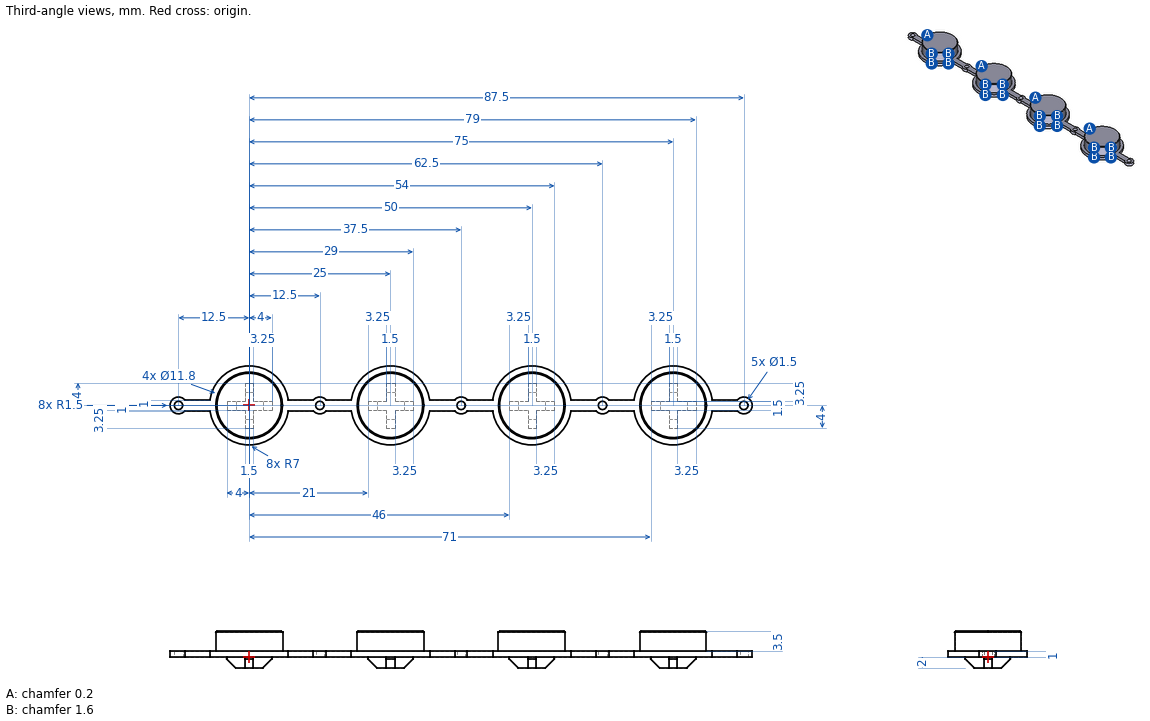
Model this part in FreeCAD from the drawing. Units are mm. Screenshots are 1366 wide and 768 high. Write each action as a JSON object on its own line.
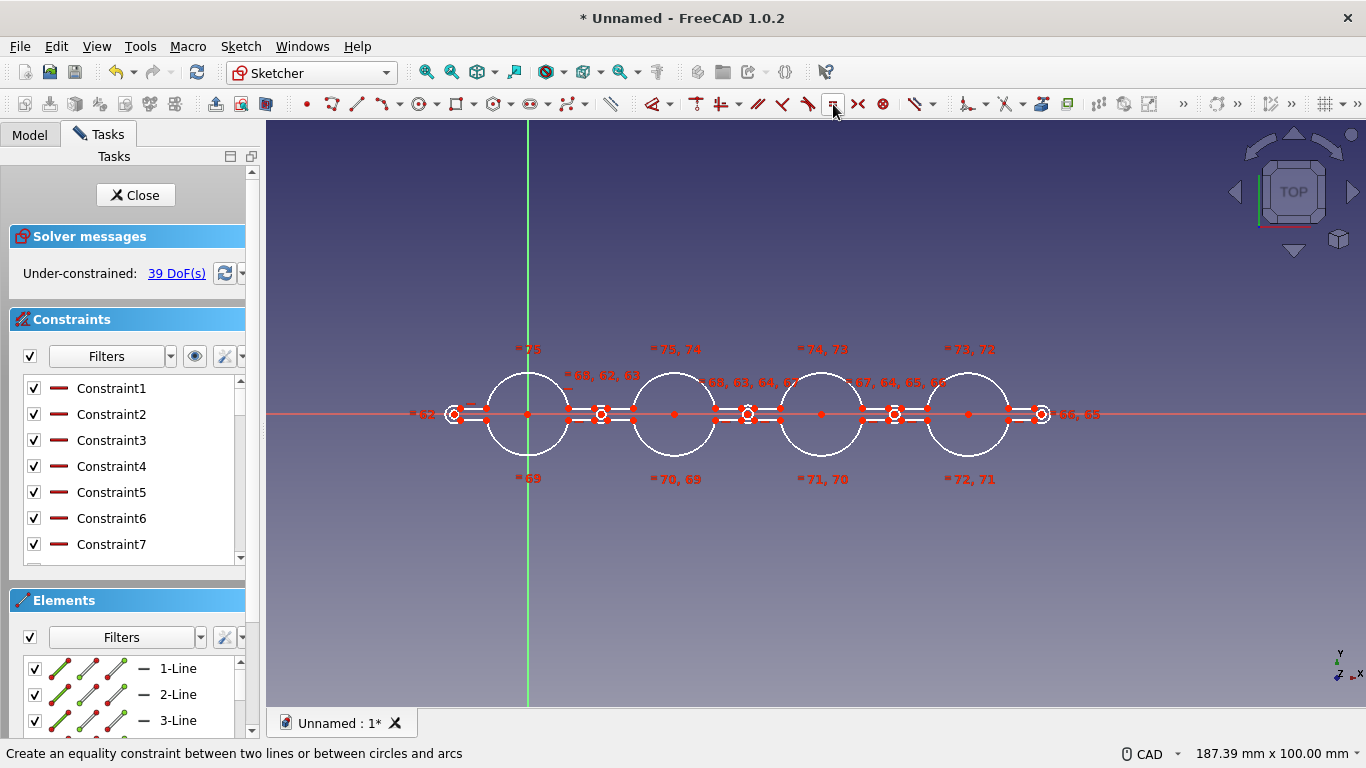
{"action": "scroll", "coordinate": [1037, 414], "scroll_direction": "up", "scroll_amount": 6}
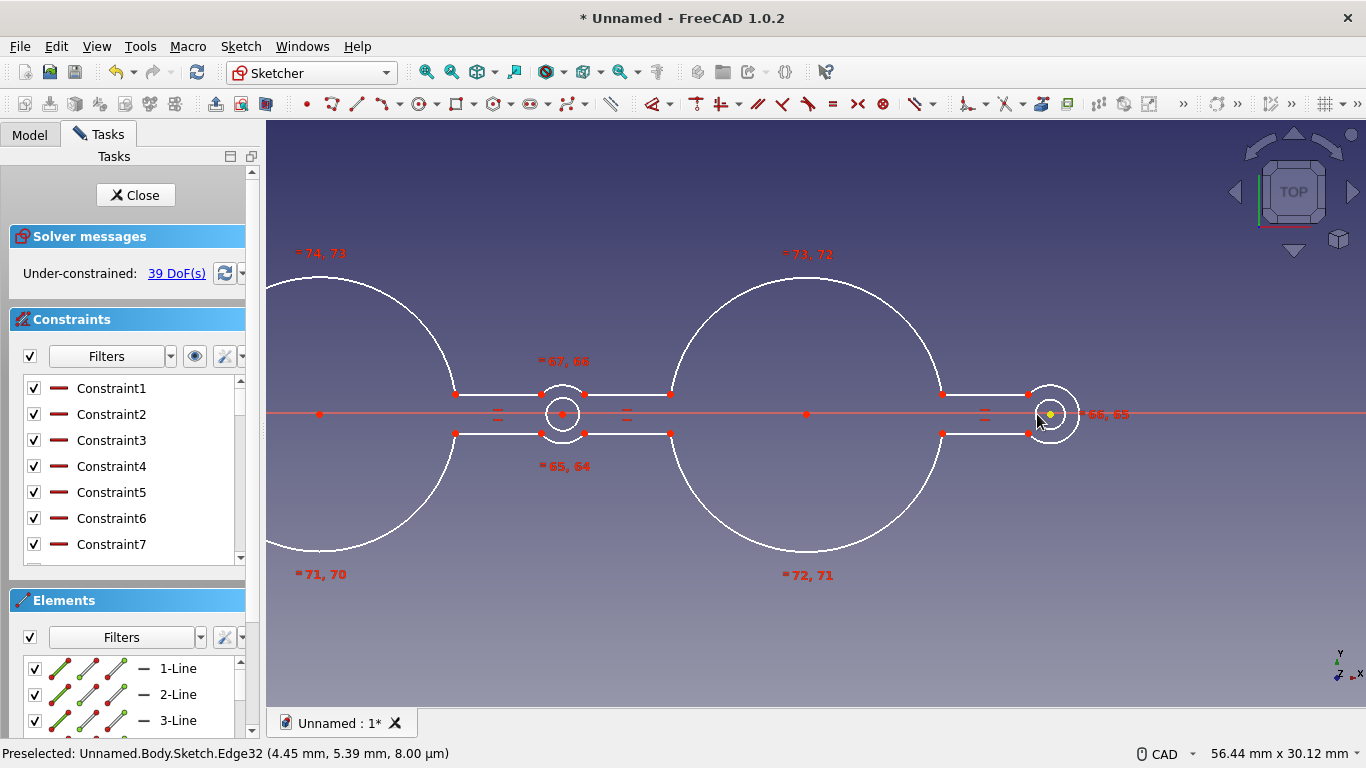
{"action": "left_click", "coordinate": [1036, 414]}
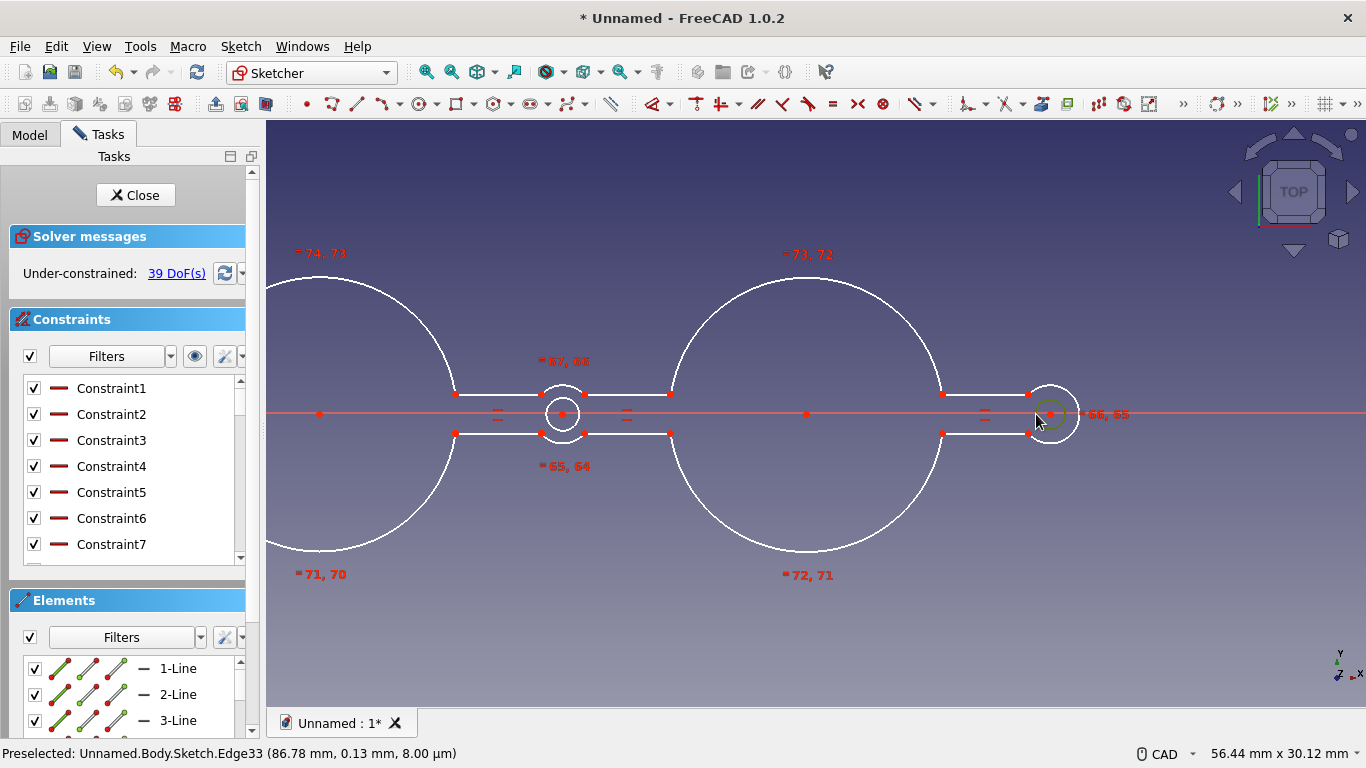
{"action": "scroll", "coordinate": [574, 403], "scroll_direction": "up", "scroll_amount": 2}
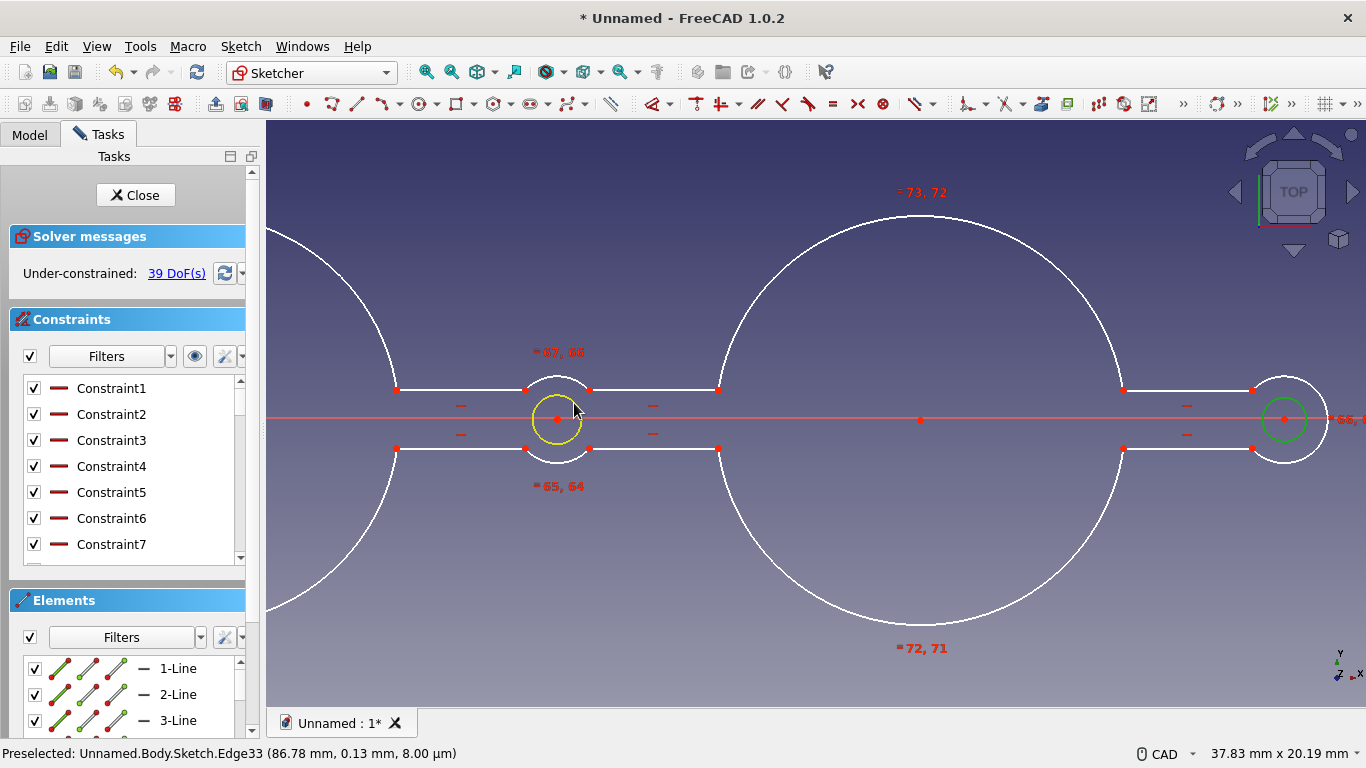
{"action": "left_click", "coordinate": [574, 402]}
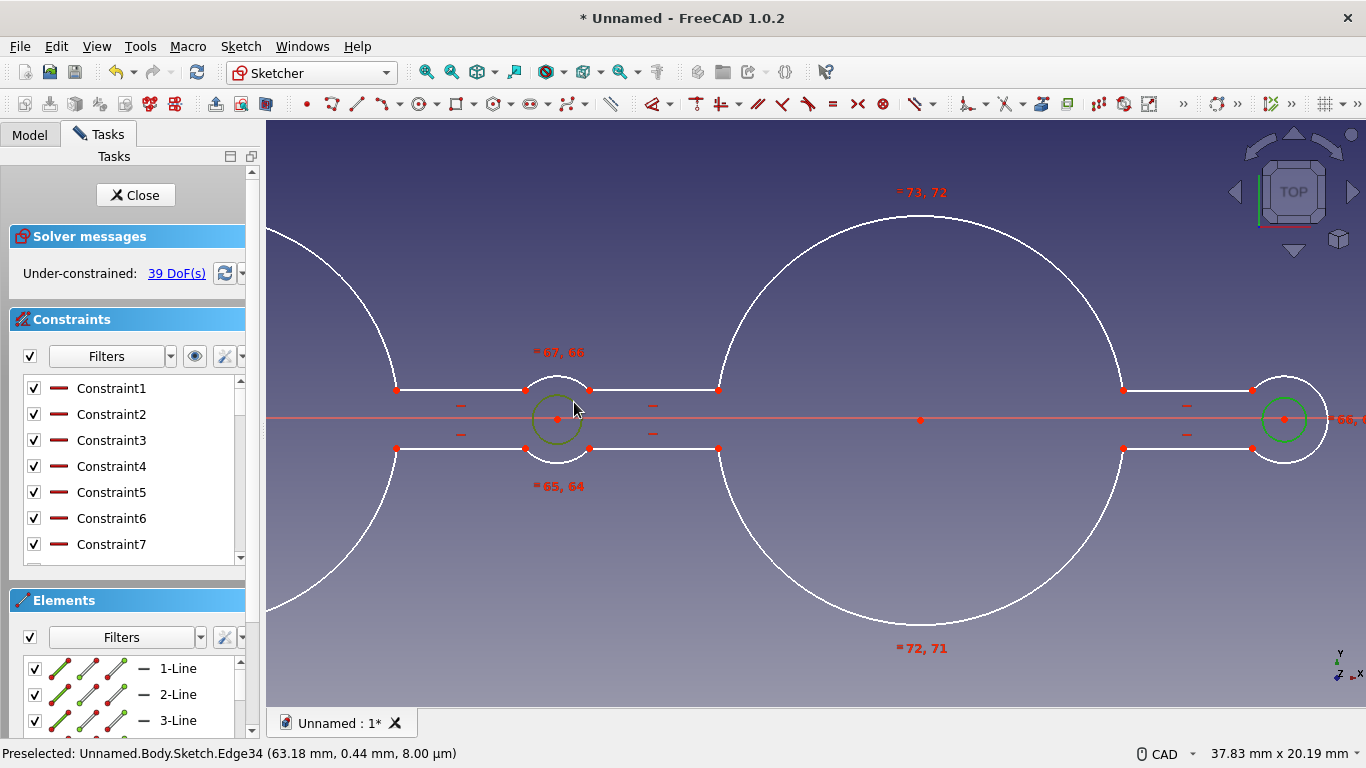
{"action": "scroll", "coordinate": [980, 412], "scroll_direction": "down", "scroll_amount": 8}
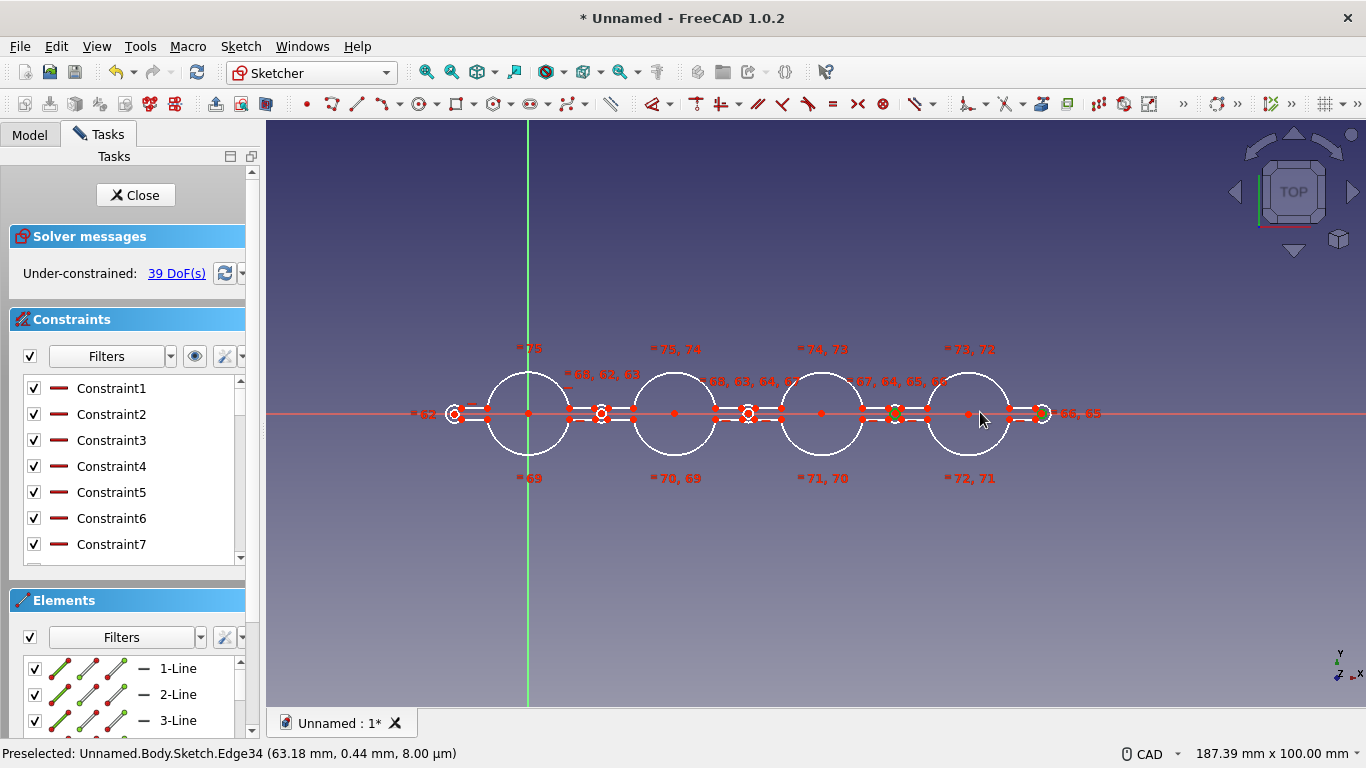
{"action": "scroll", "coordinate": [752, 410], "scroll_direction": "up", "scroll_amount": 7}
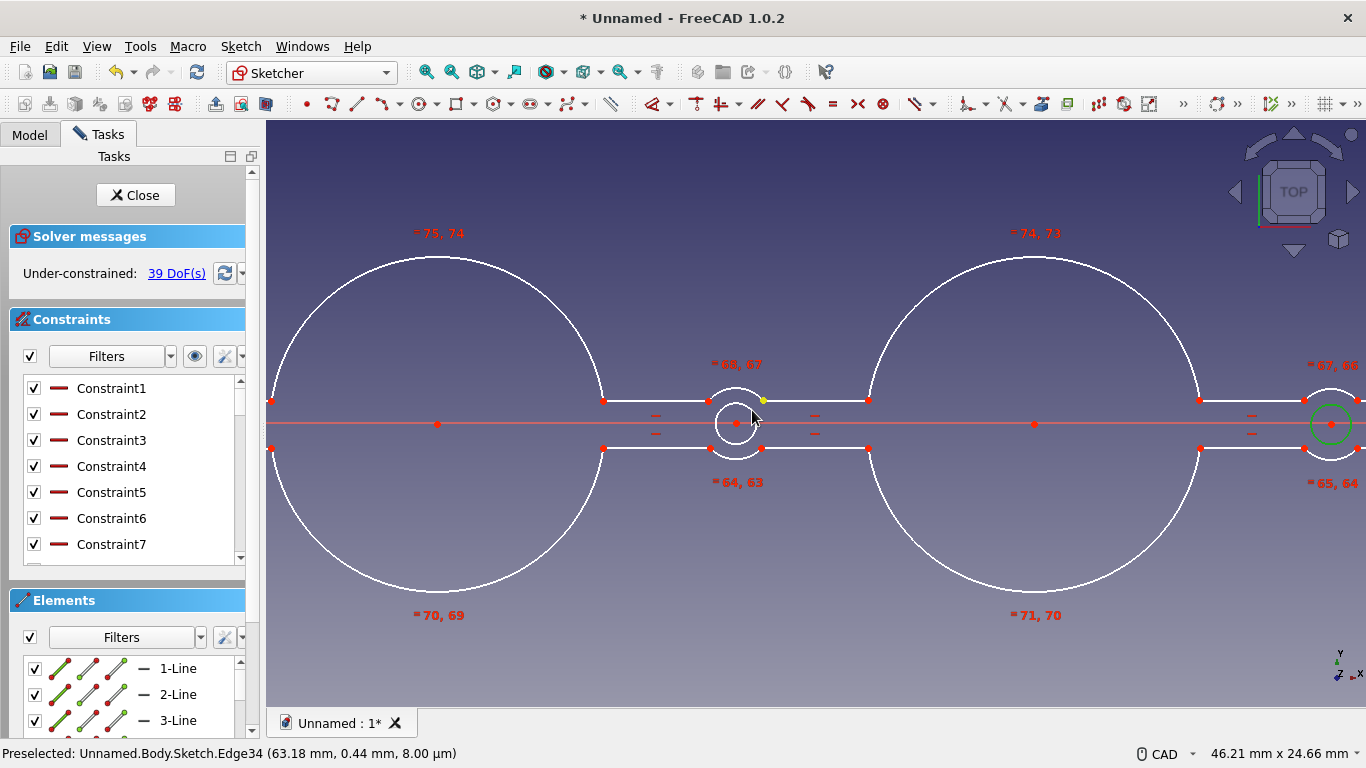
{"action": "left_click", "coordinate": [750, 409]}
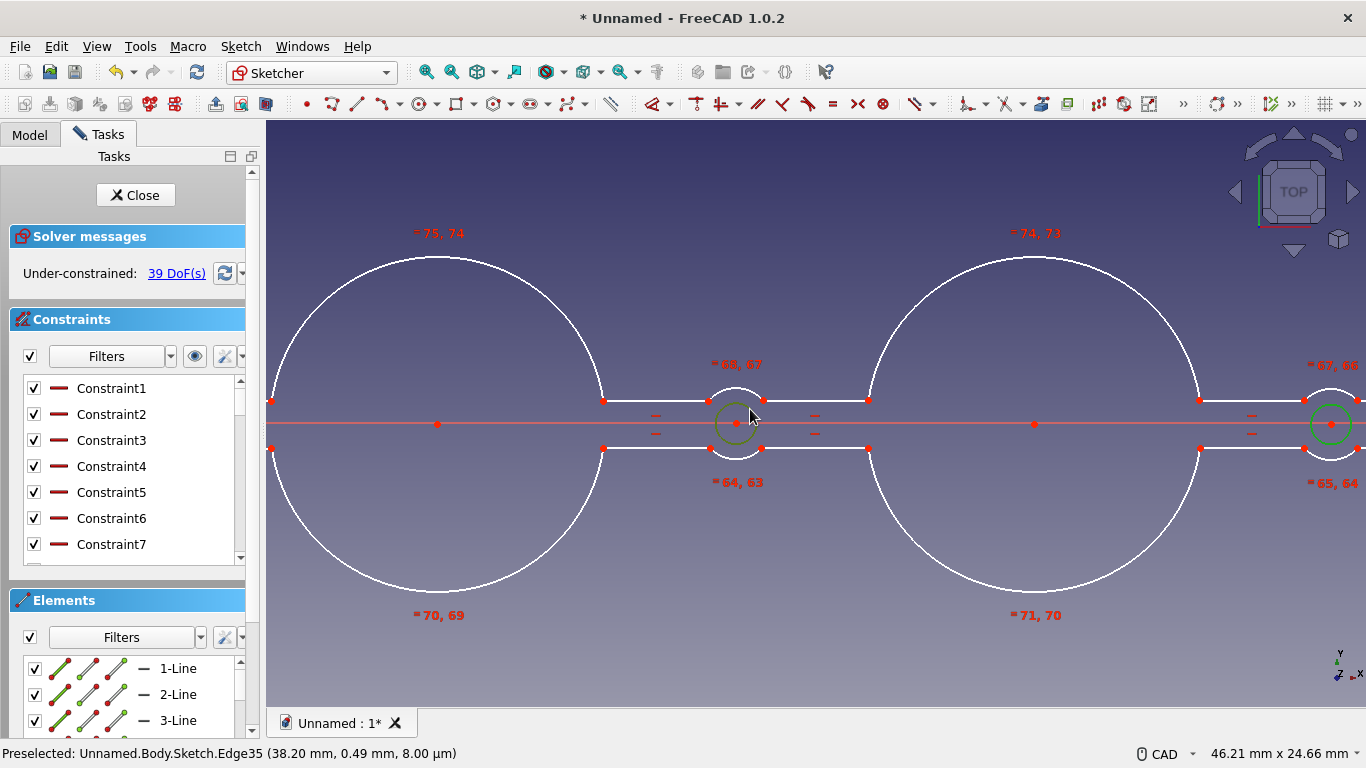
{"action": "scroll", "coordinate": [751, 410], "scroll_direction": "down", "scroll_amount": 7}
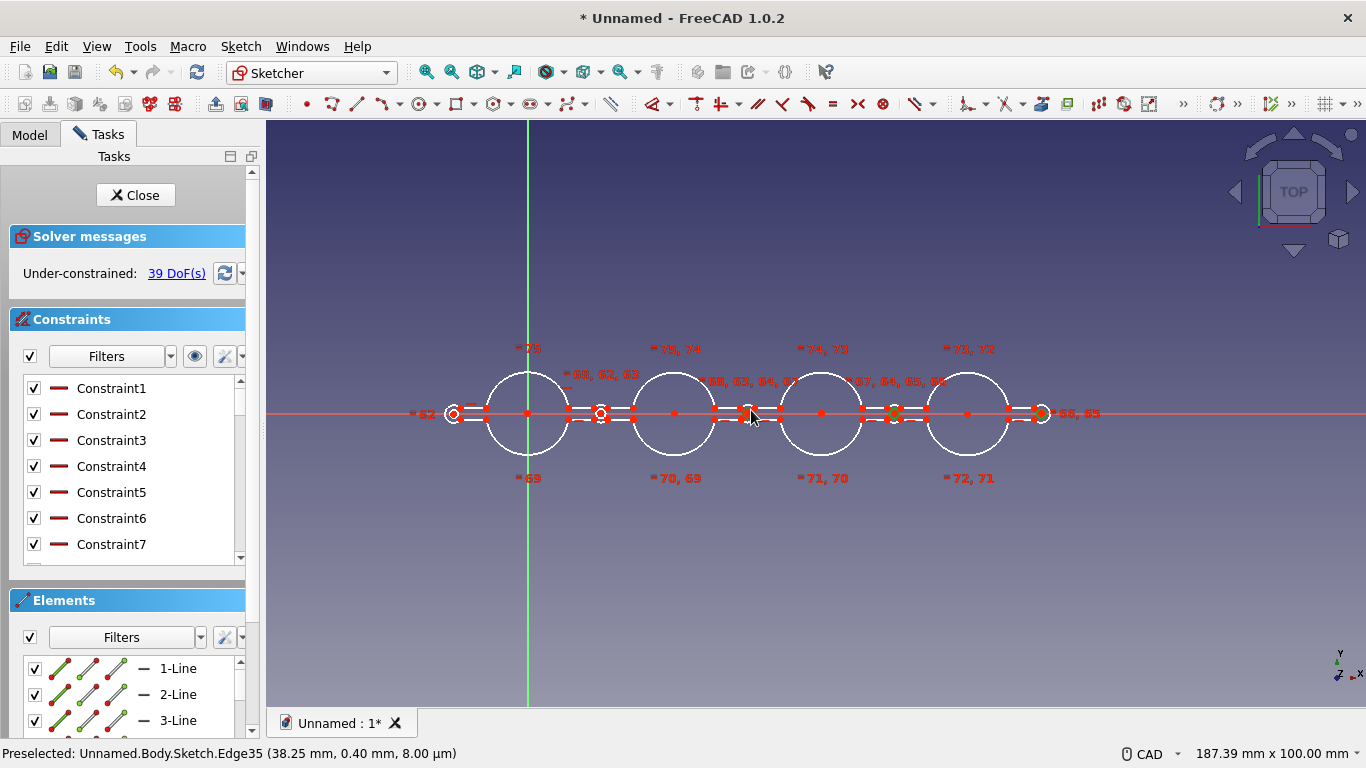
{"action": "scroll", "coordinate": [604, 411], "scroll_direction": "up", "scroll_amount": 8}